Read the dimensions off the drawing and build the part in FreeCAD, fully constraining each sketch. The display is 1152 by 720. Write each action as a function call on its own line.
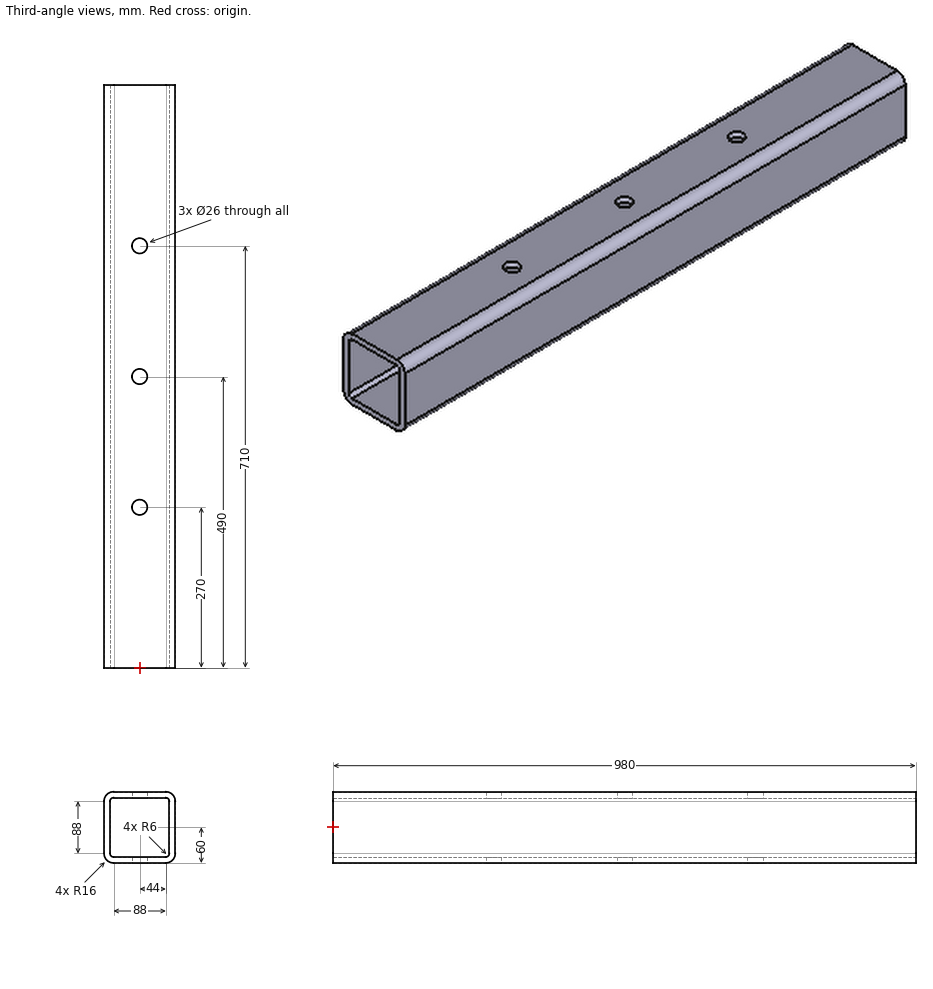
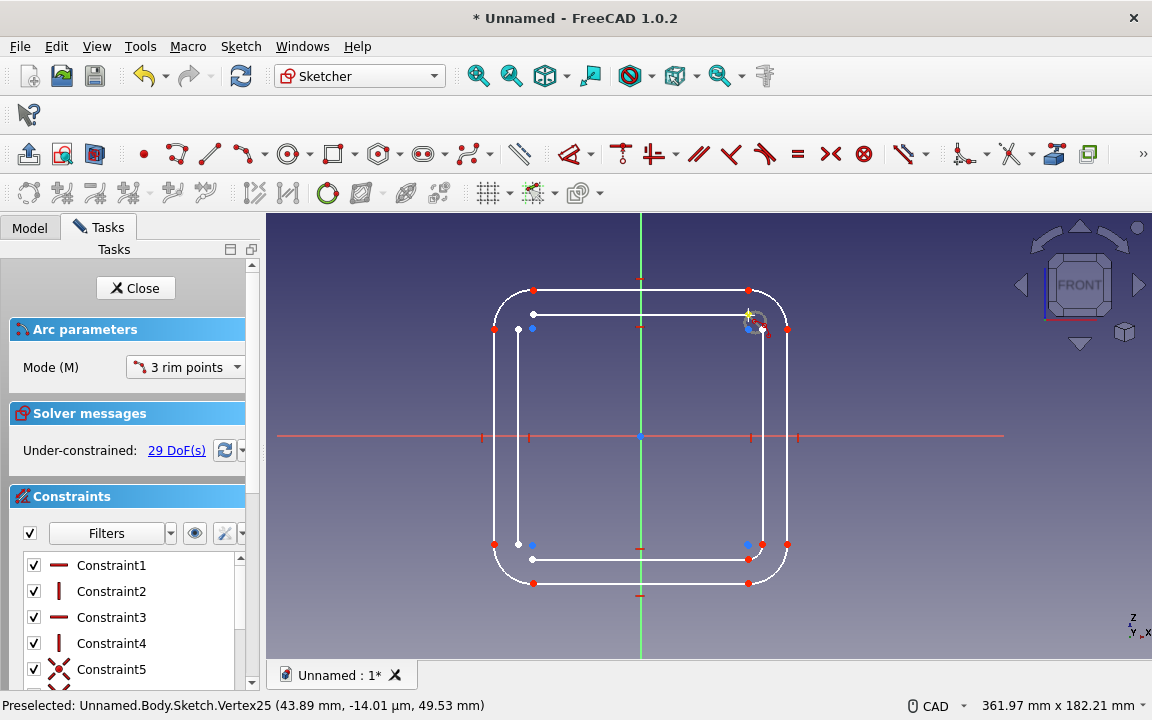
scroll(759, 318, up, 7)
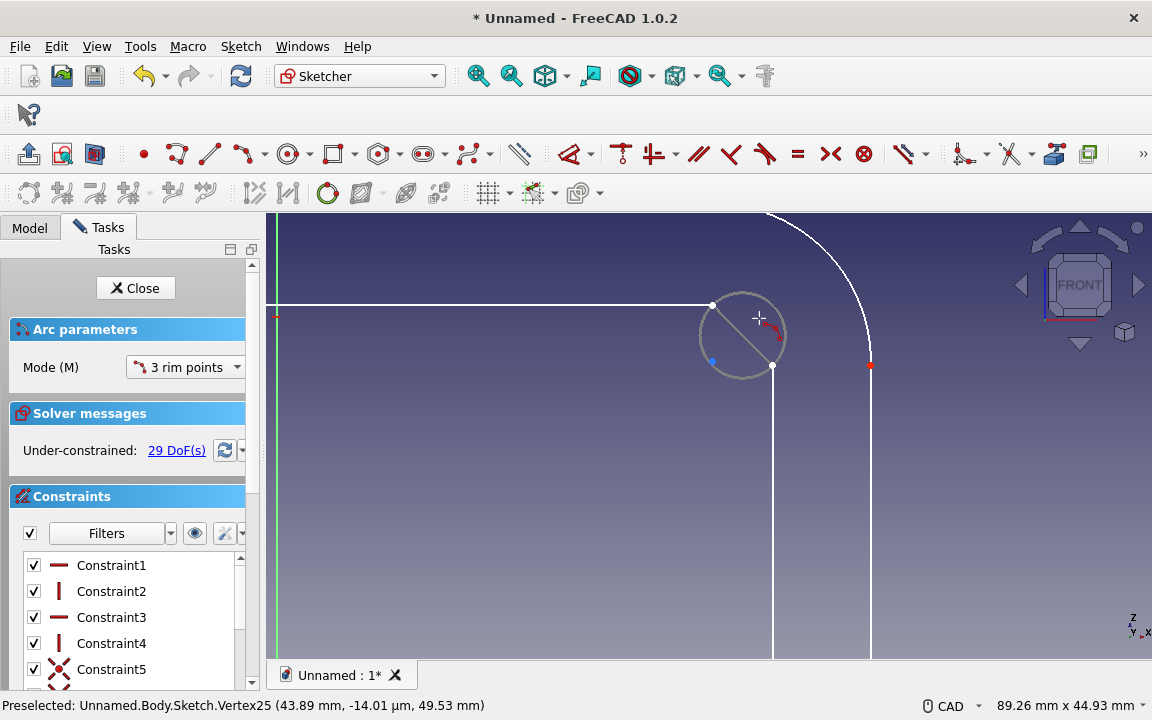
click(756, 318)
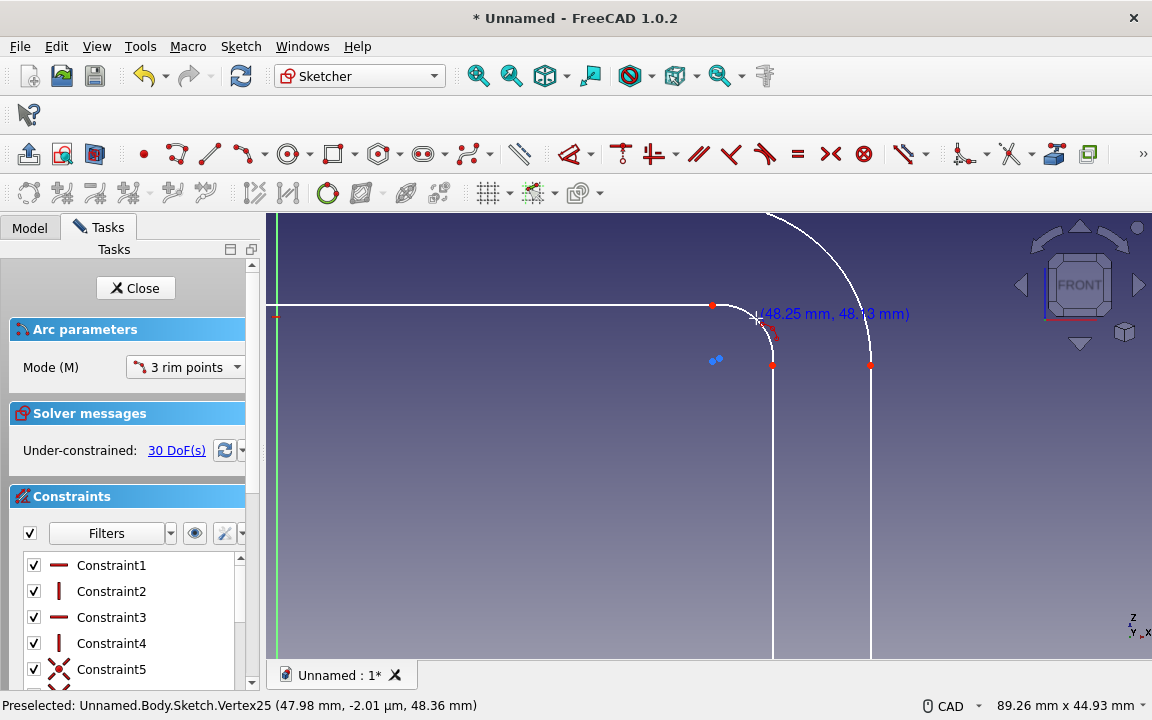
scroll(759, 318, down, 7)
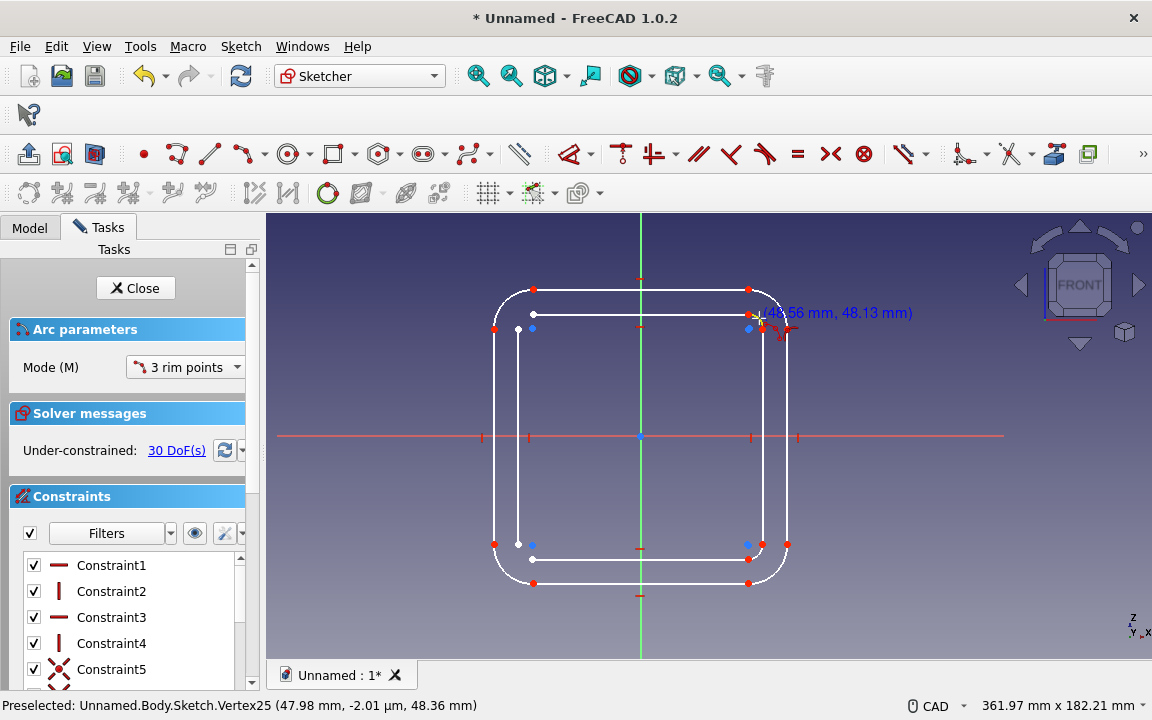
click(533, 315)
click(518, 330)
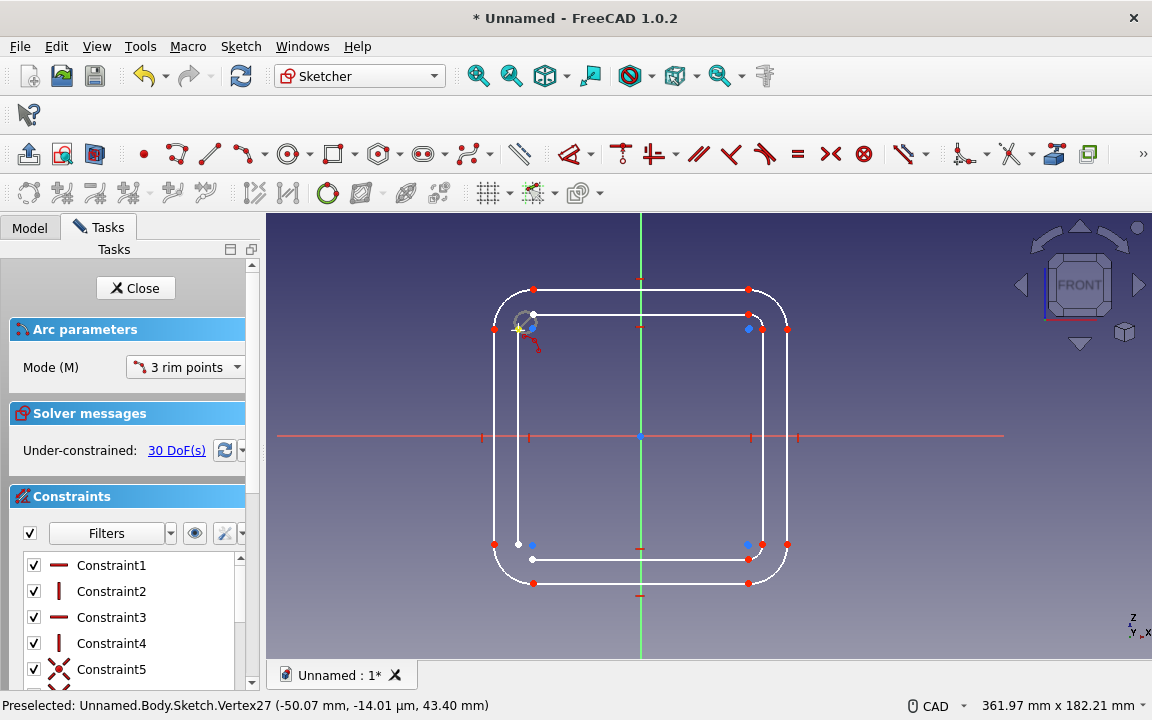
scroll(522, 318, up, 7)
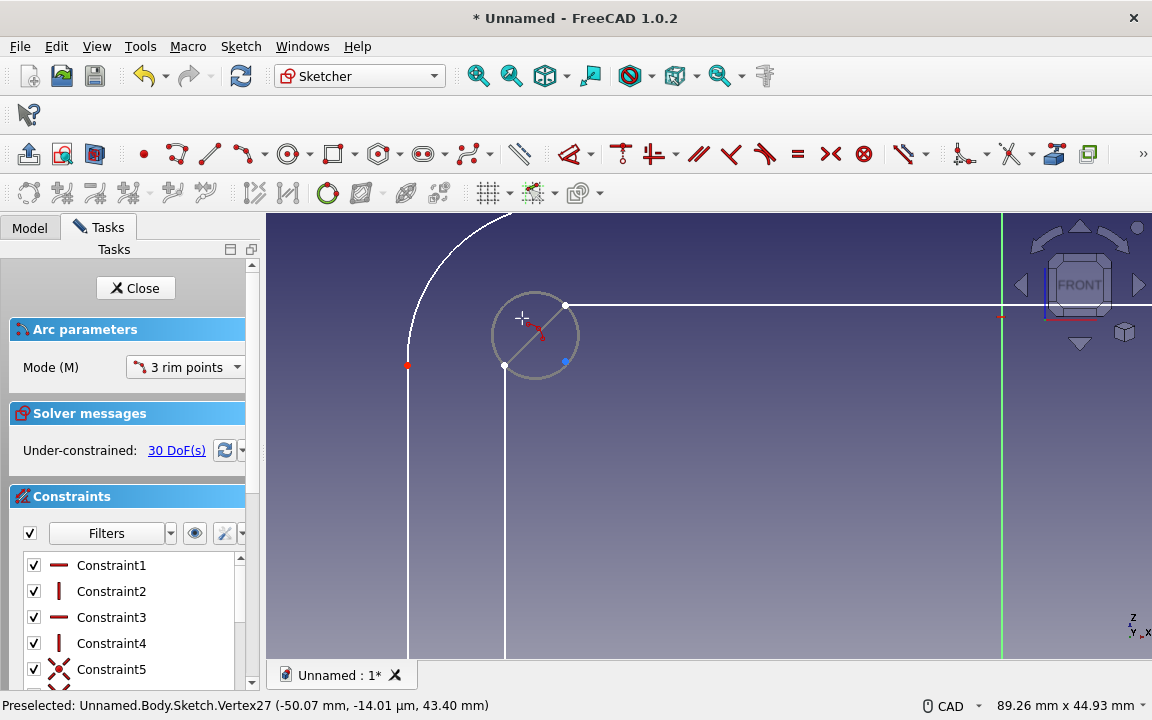
click(523, 318)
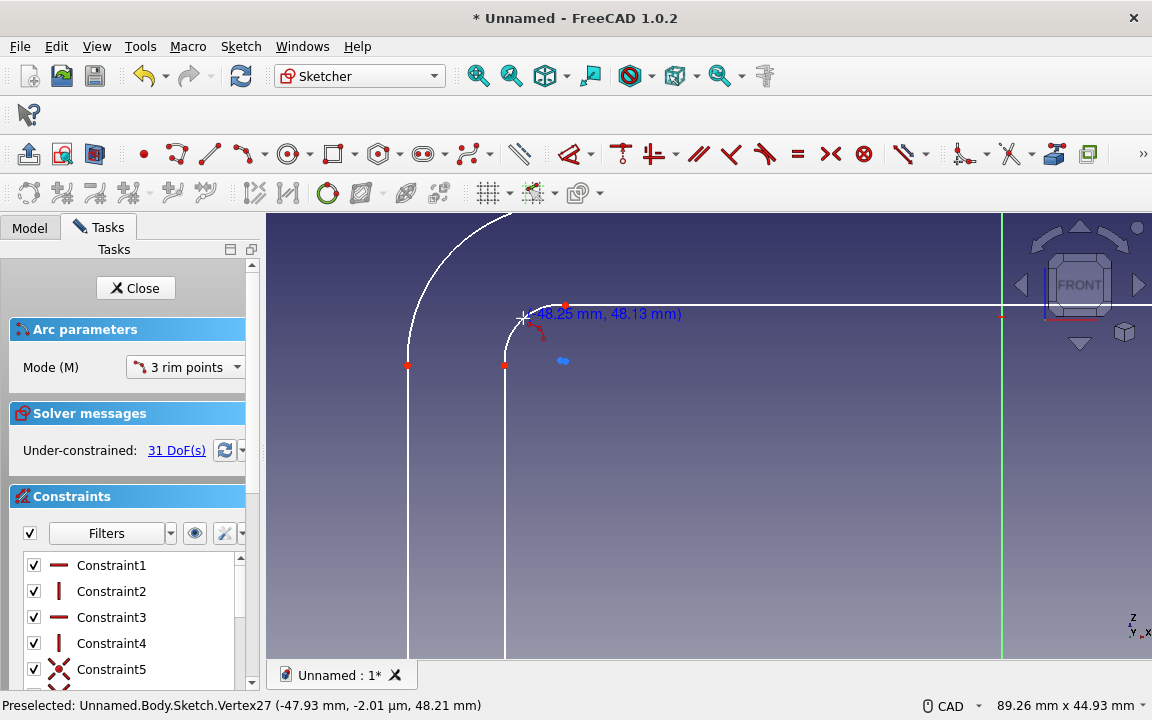
scroll(522, 318, down, 7)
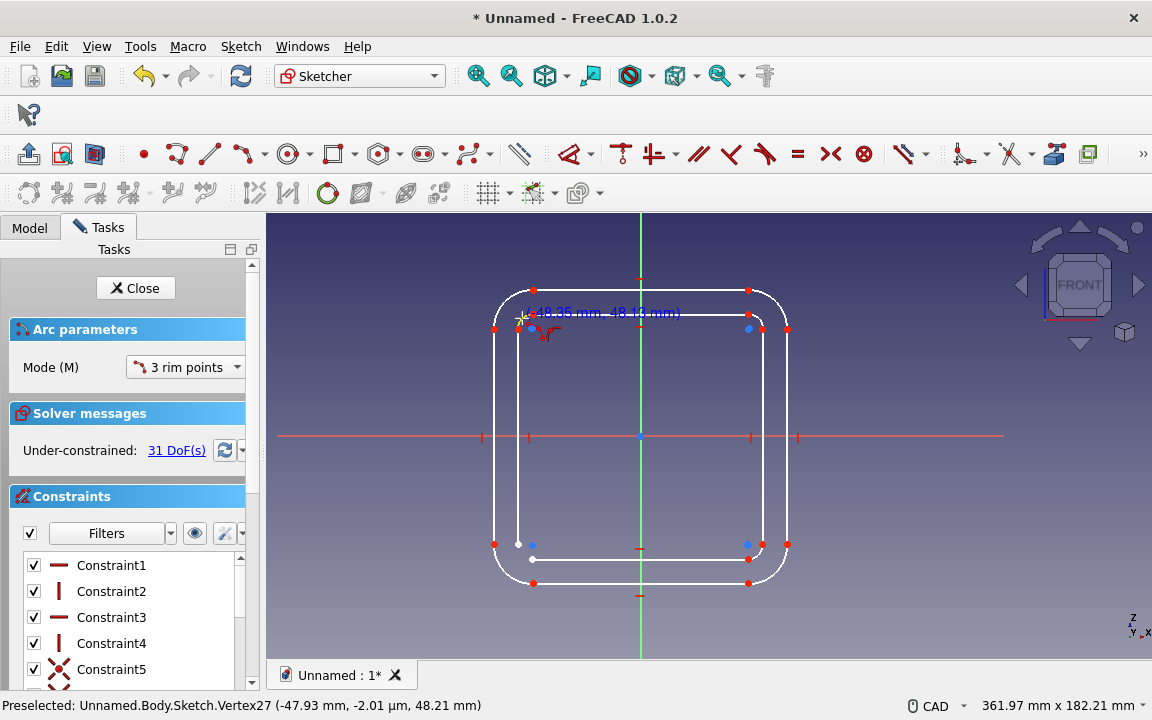
click(518, 545)
click(533, 560)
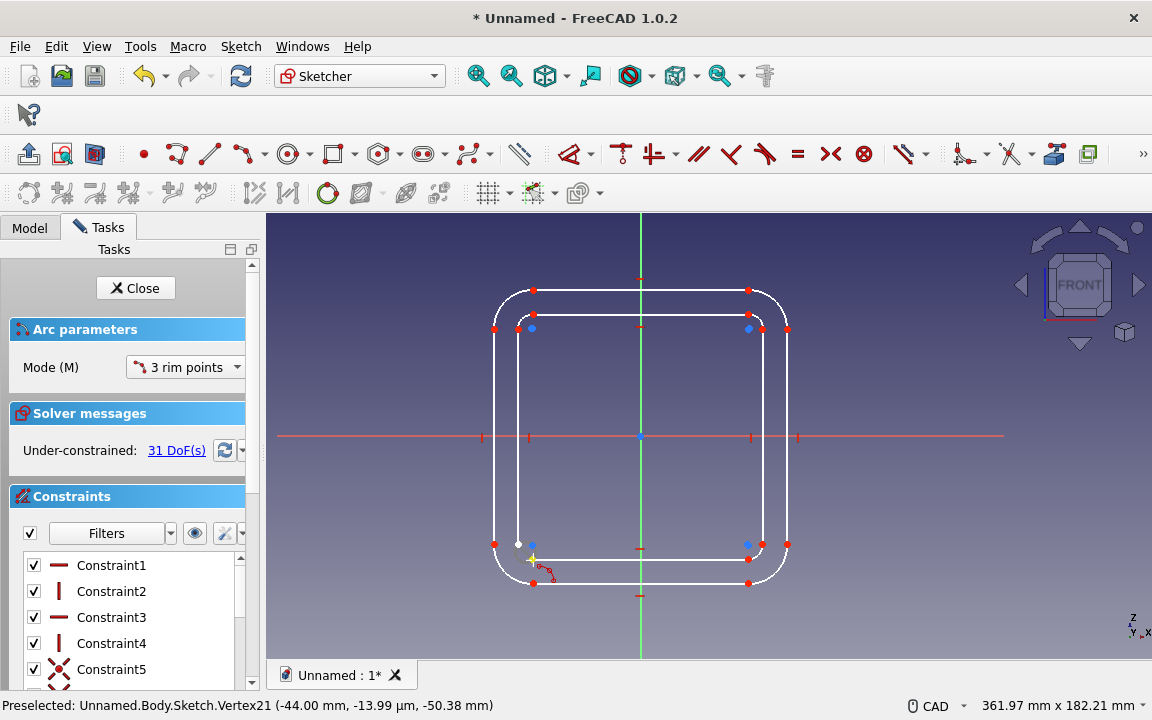
scroll(522, 554, up, 7)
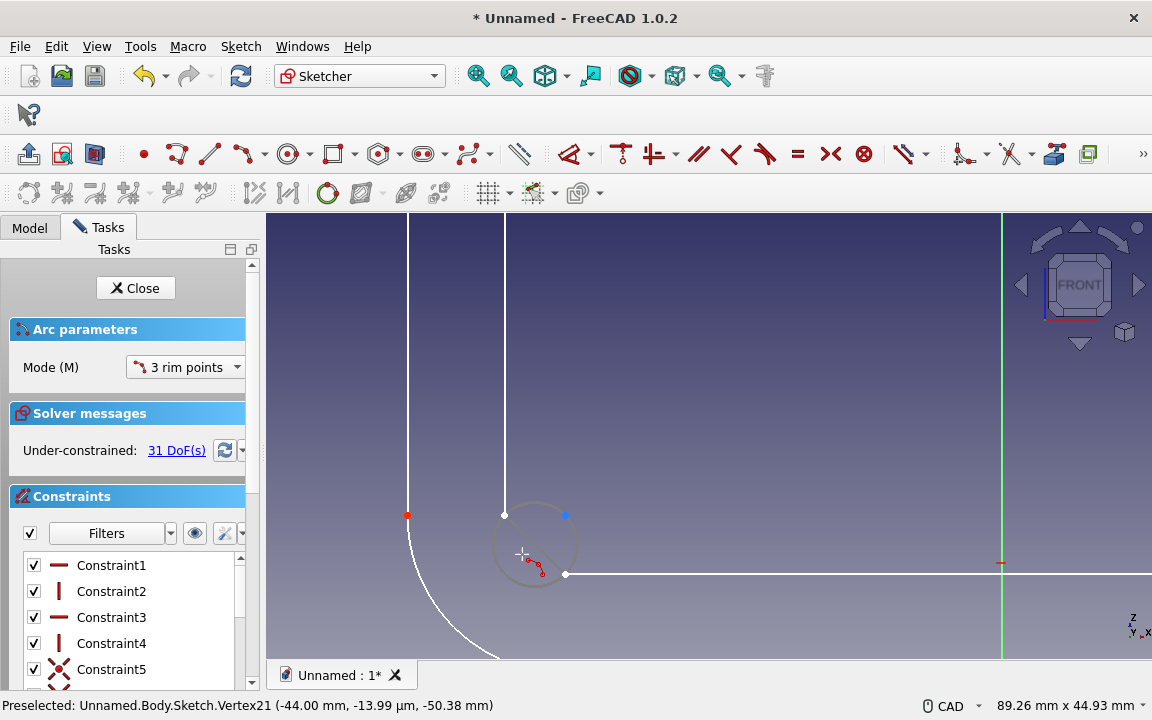
click(523, 553)
key(Escape)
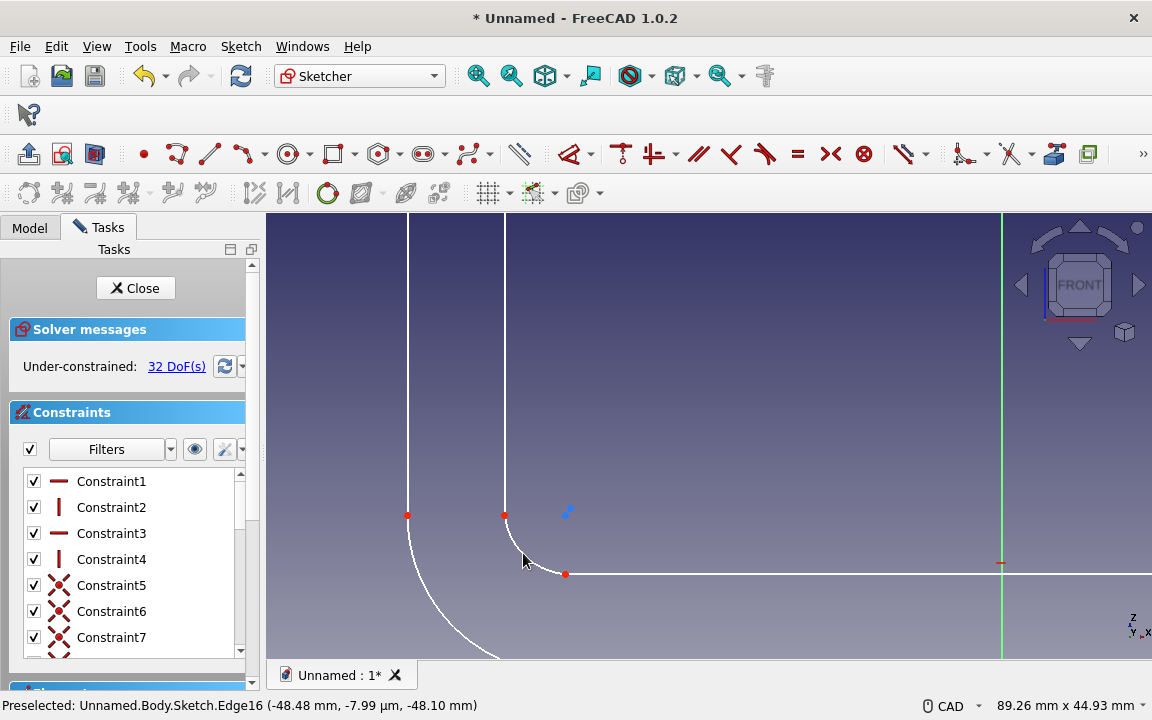
scroll(522, 554, down, 7)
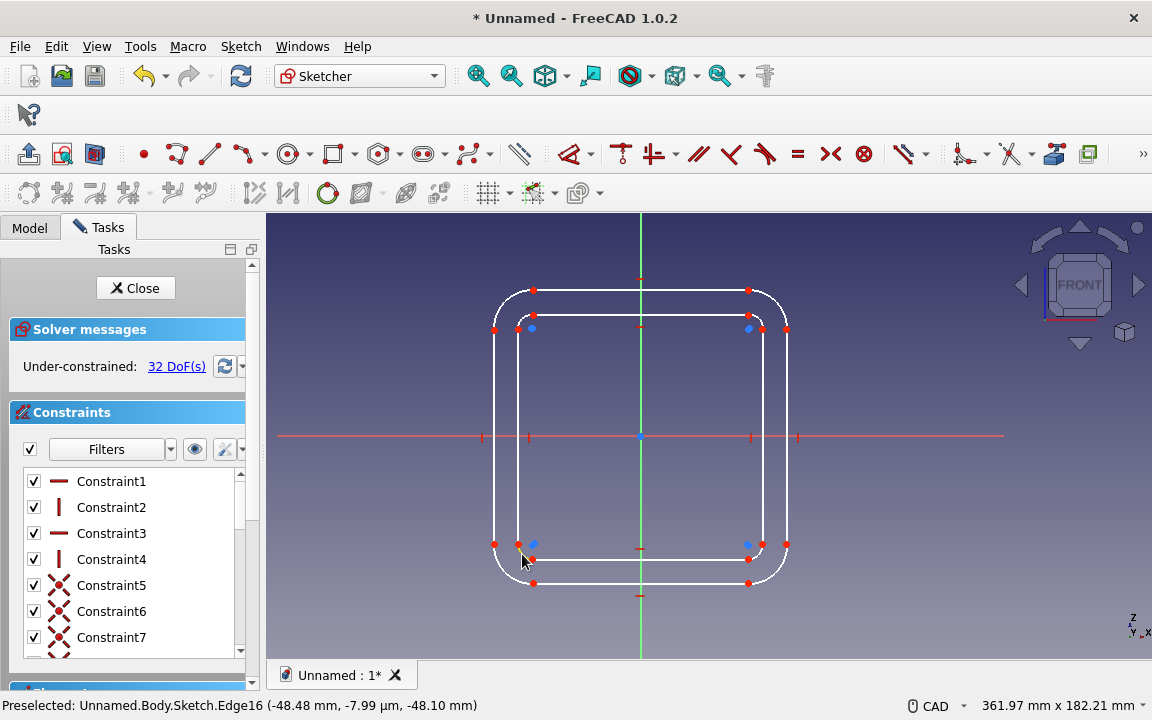
click(683, 584)